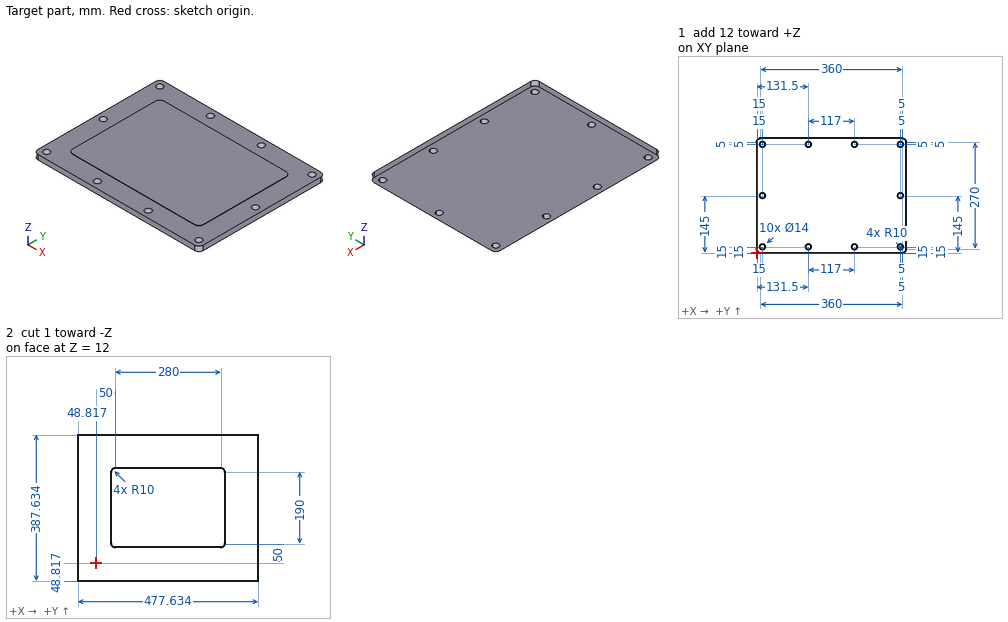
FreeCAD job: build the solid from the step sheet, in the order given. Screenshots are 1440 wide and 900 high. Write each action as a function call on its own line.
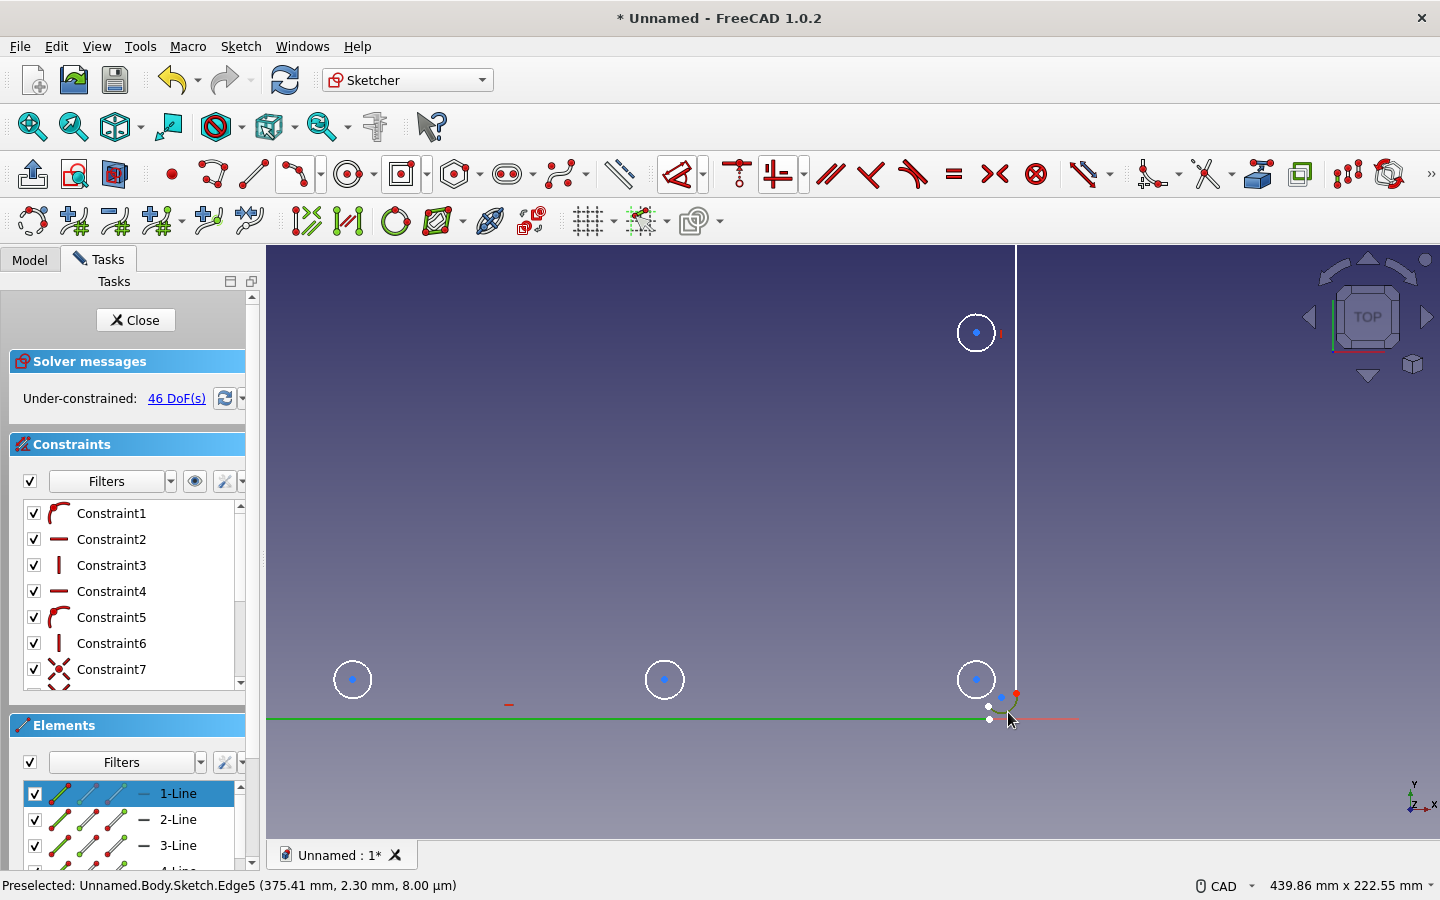
click(913, 174)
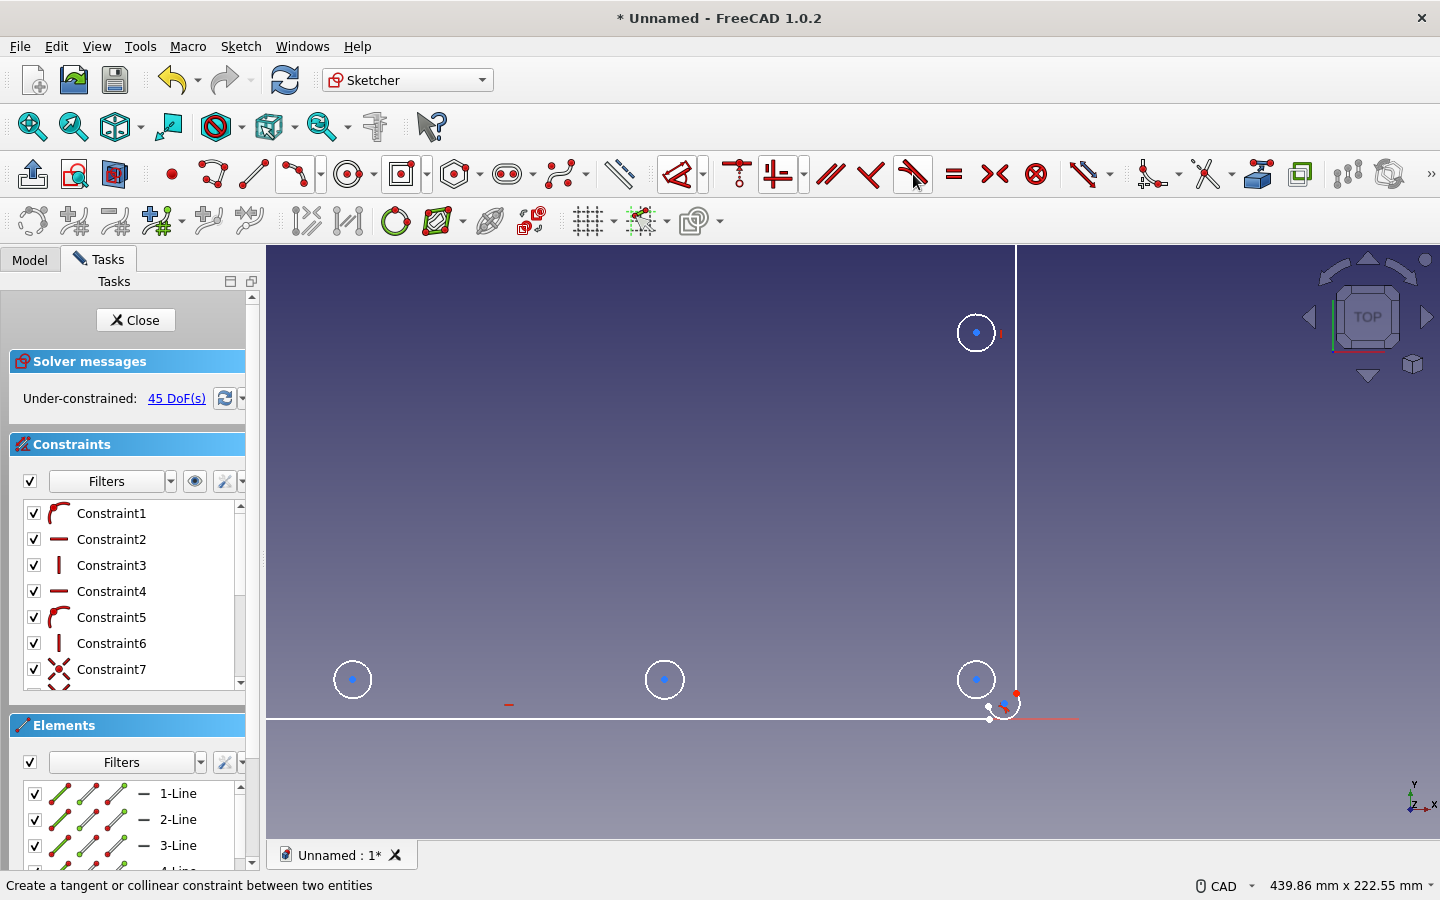
click(317, 719)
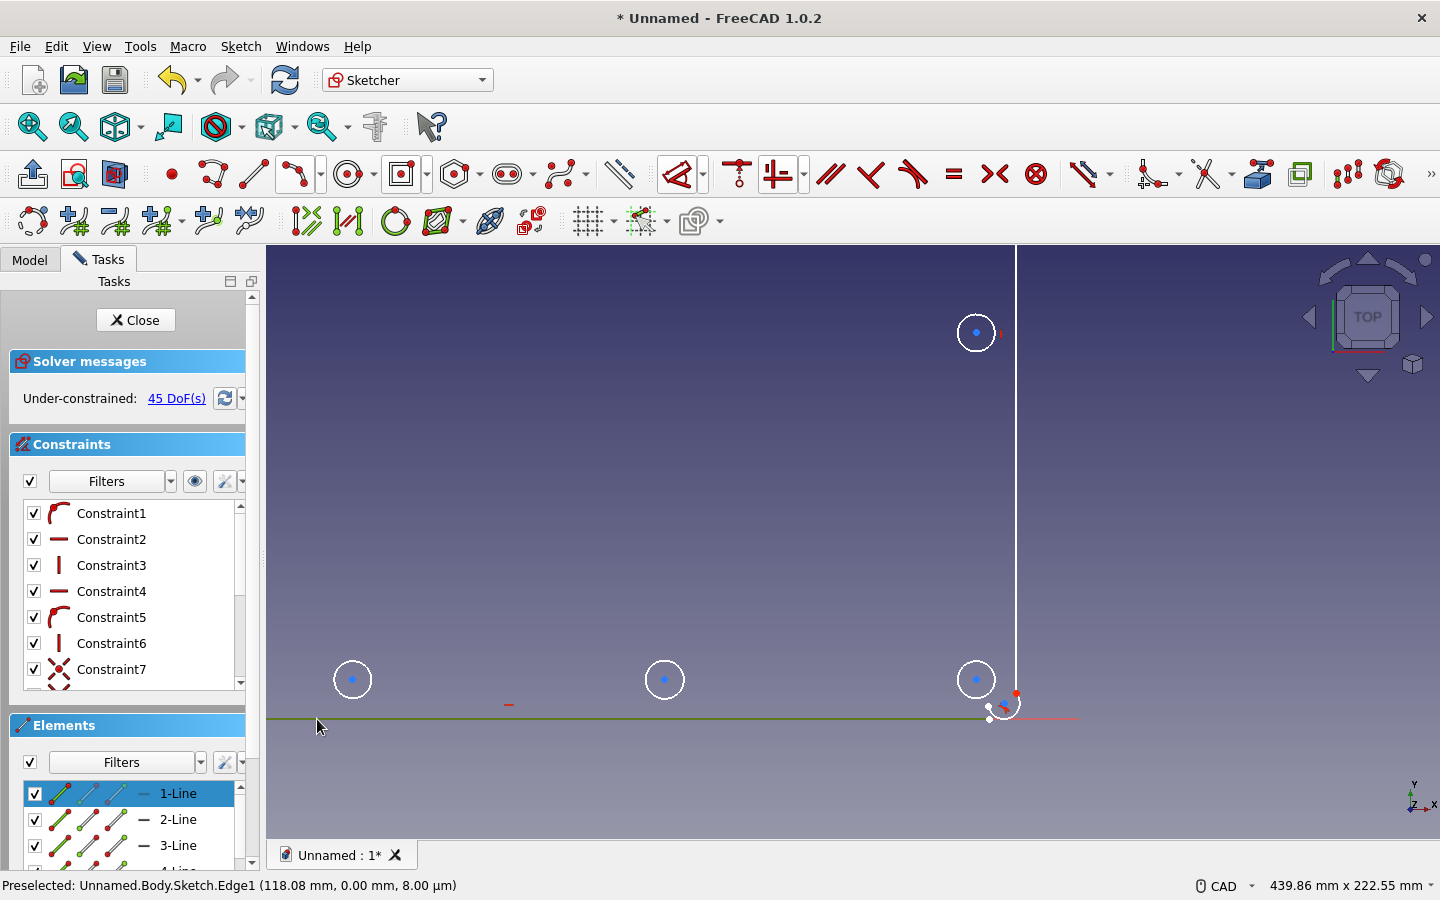
scroll(1009, 713, down, 4)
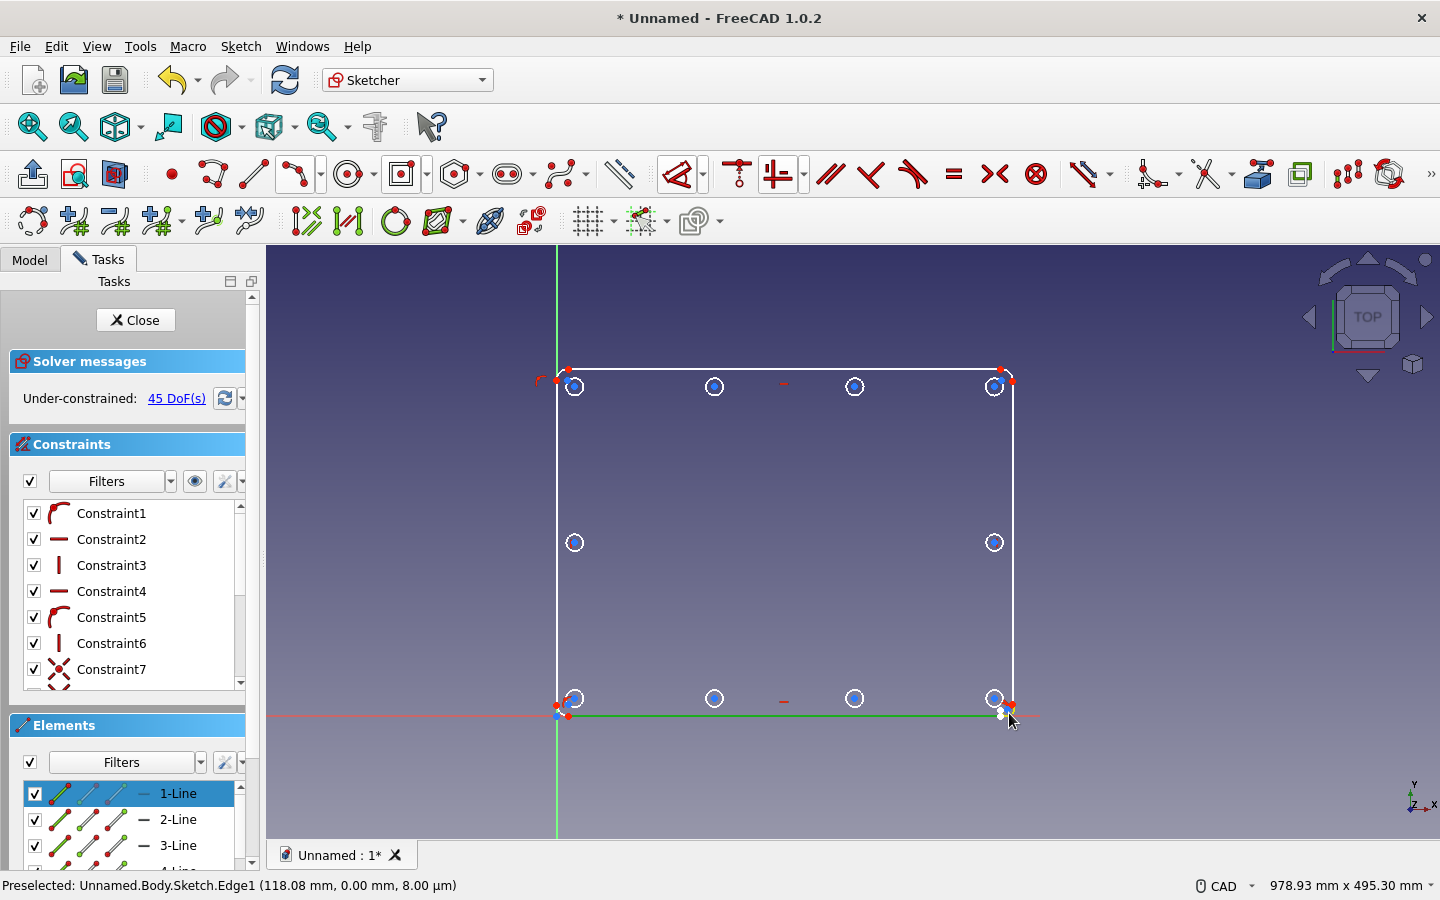
scroll(558, 710, up, 5)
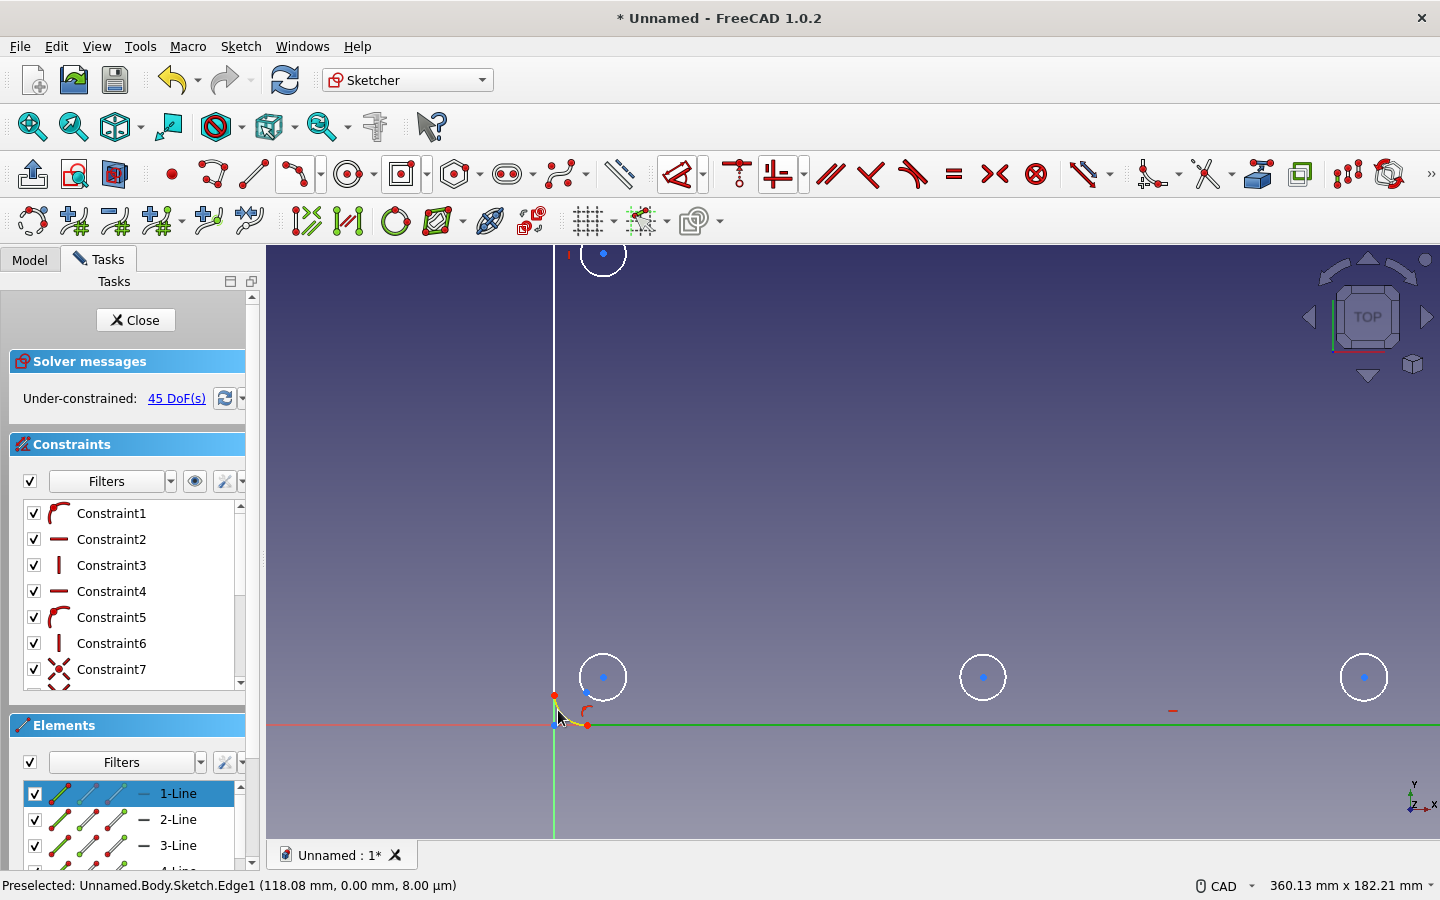
click(559, 709)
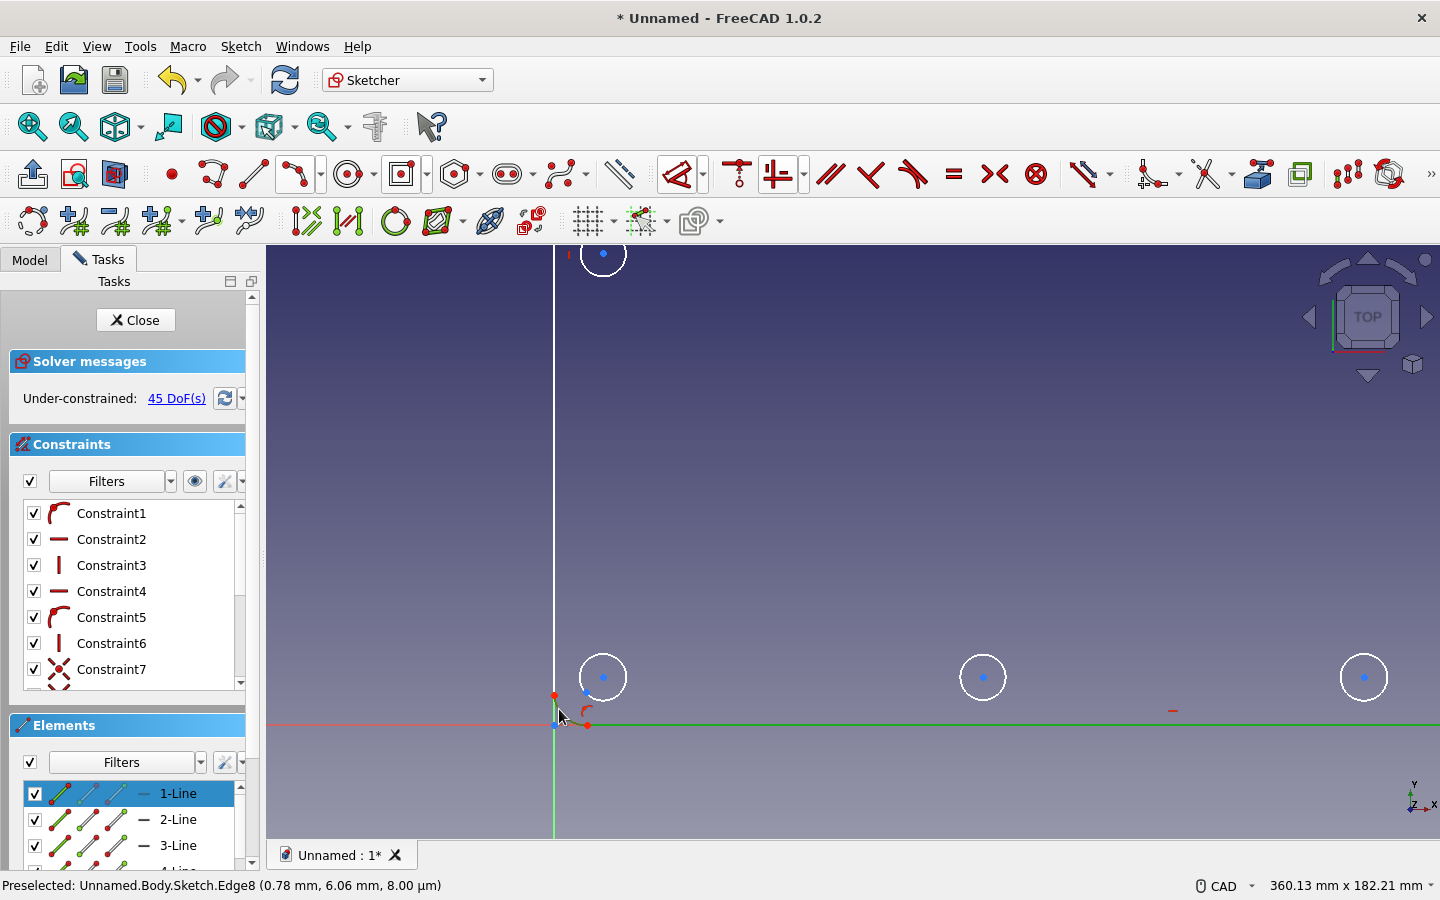
click(913, 174)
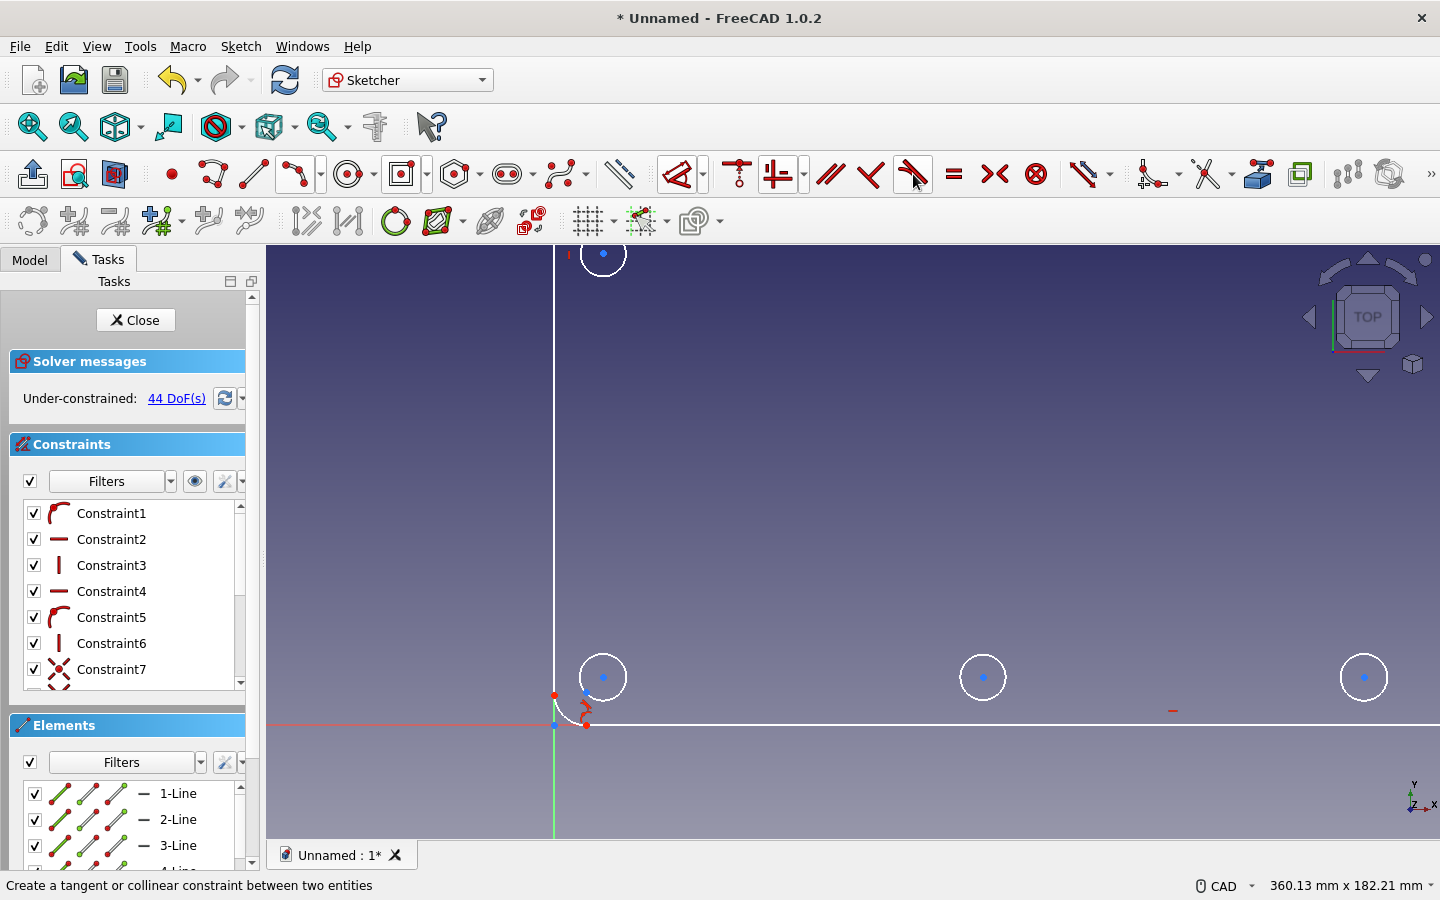
scroll(558, 710, down, 5)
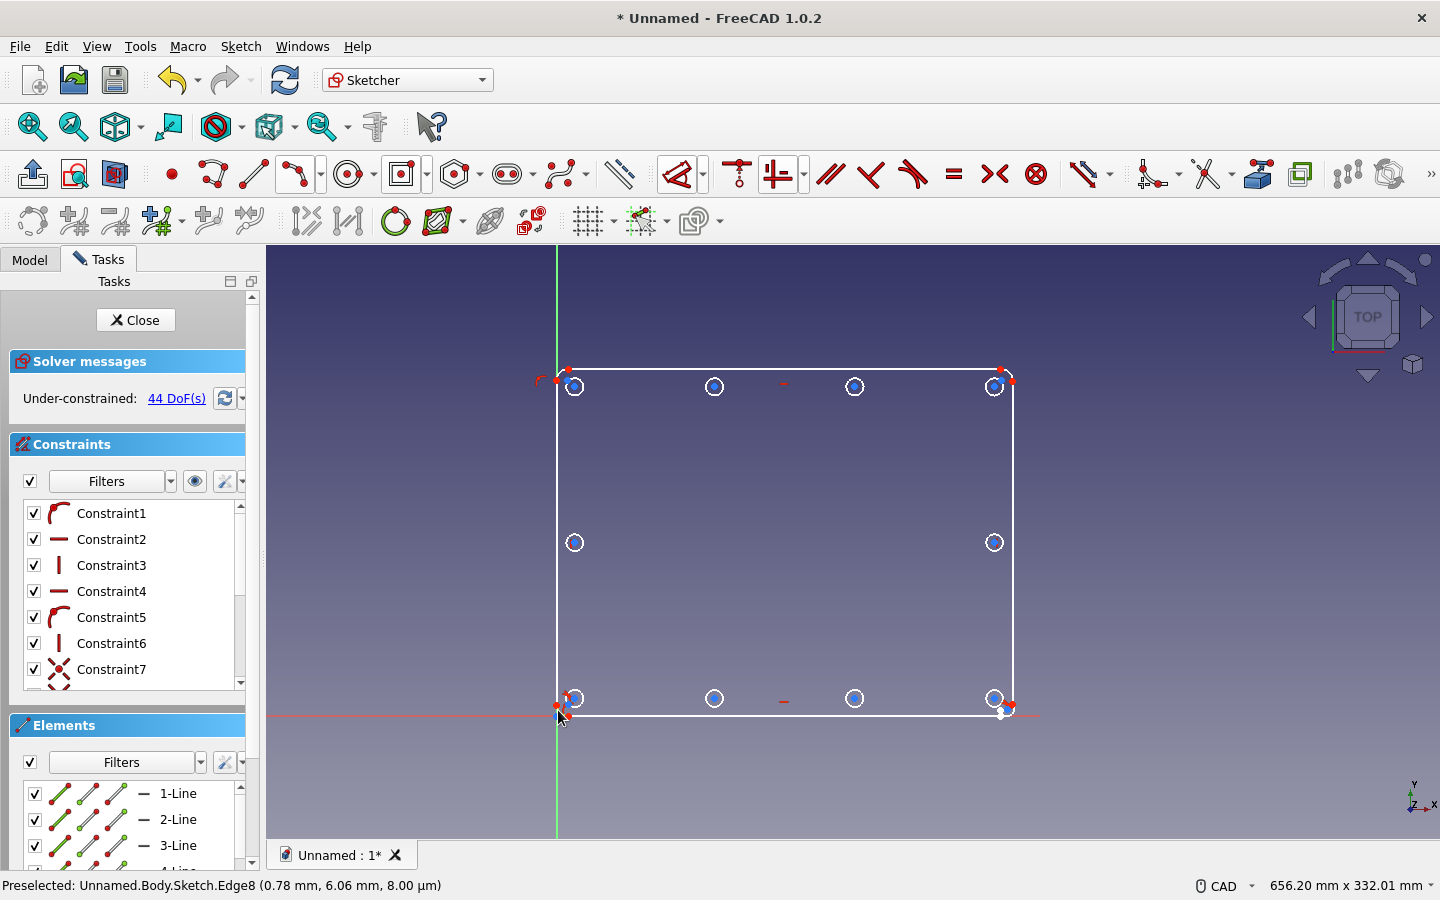
click(1013, 608)